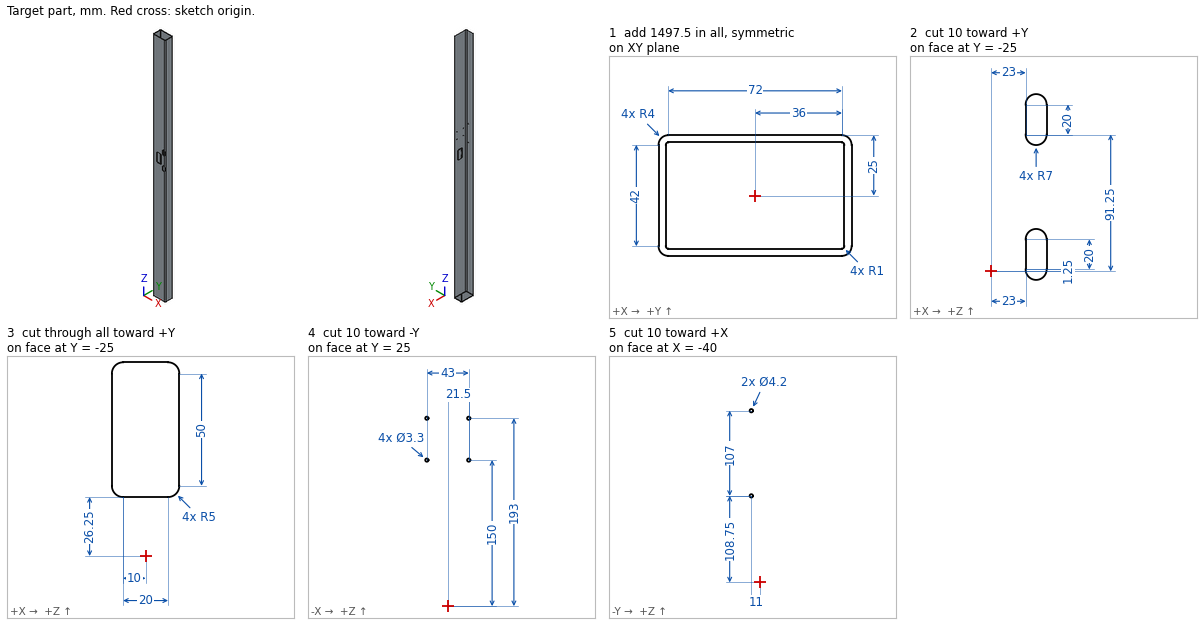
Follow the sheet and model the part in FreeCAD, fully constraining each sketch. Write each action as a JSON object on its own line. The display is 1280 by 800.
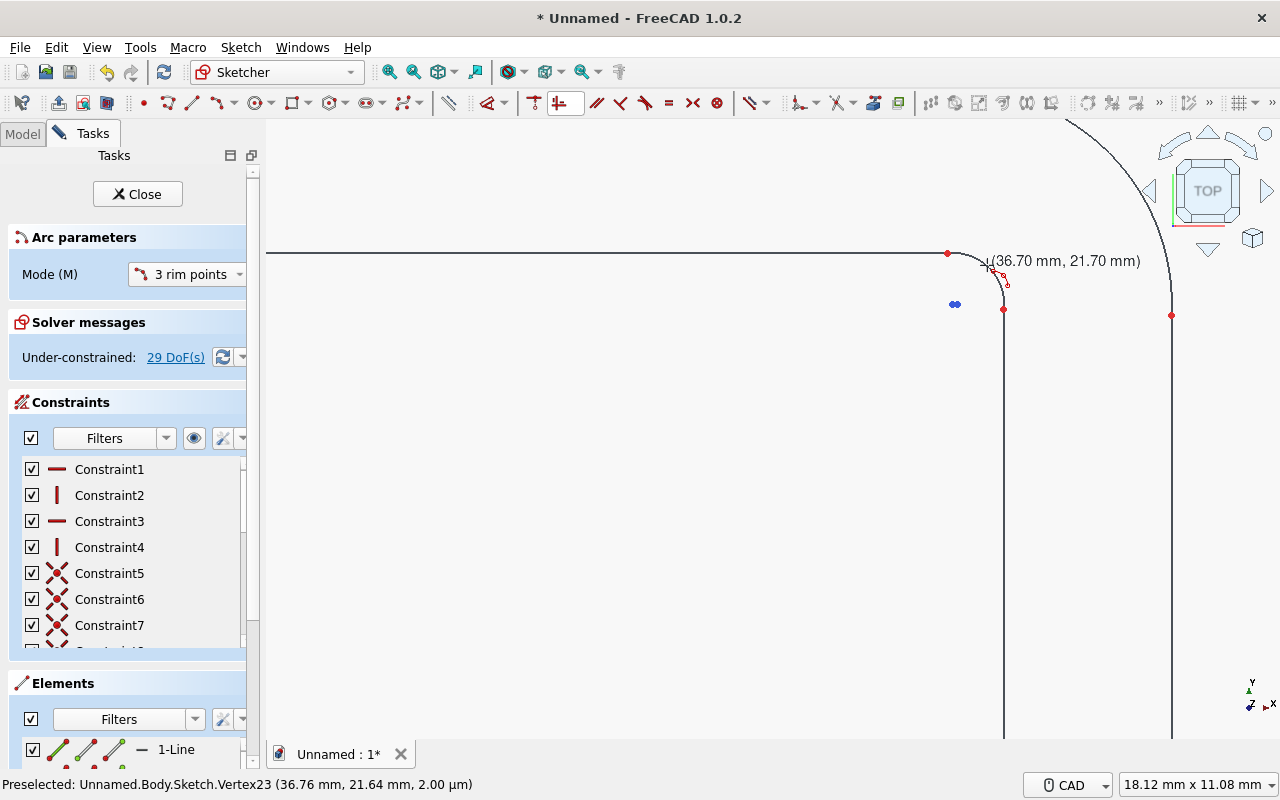
{"action": "scroll", "coordinate": [982, 264], "scroll_direction": "down", "scroll_amount": 10}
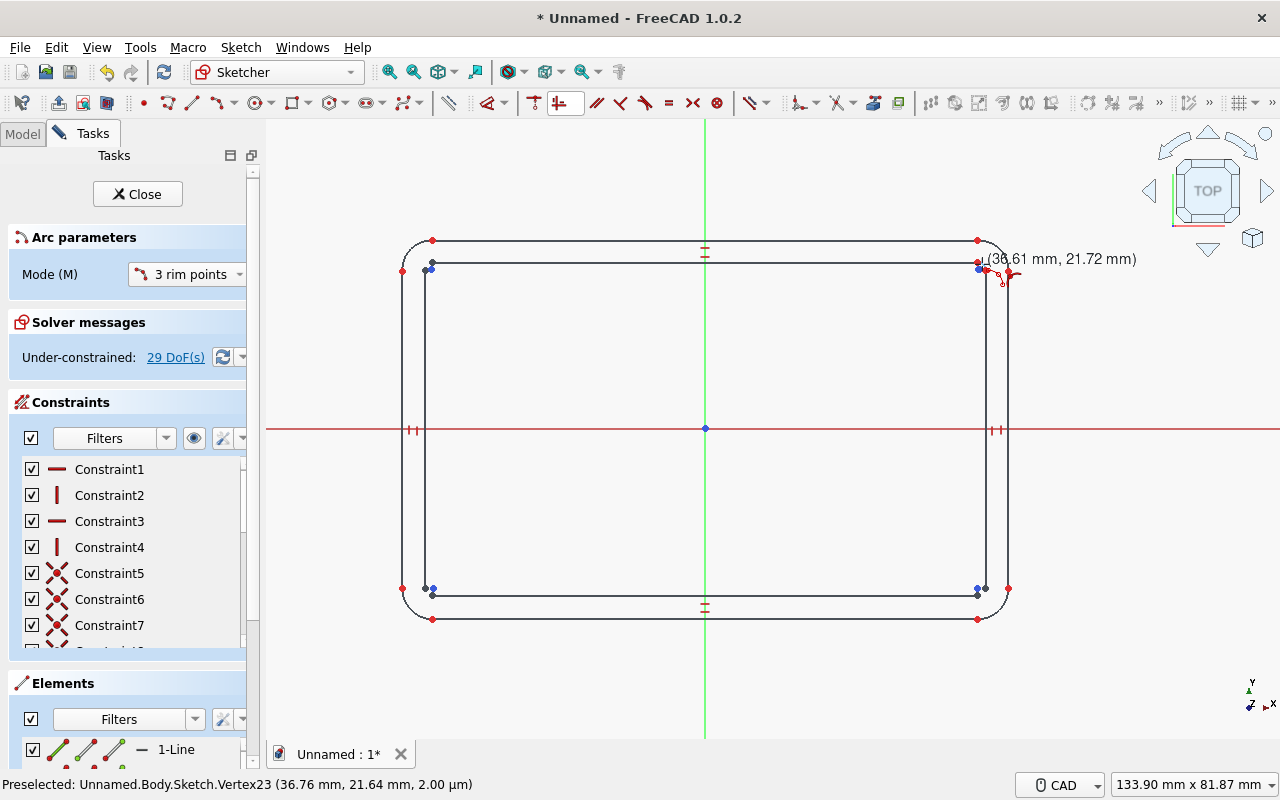
{"action": "scroll", "coordinate": [986, 588], "scroll_direction": "up", "scroll_amount": 4}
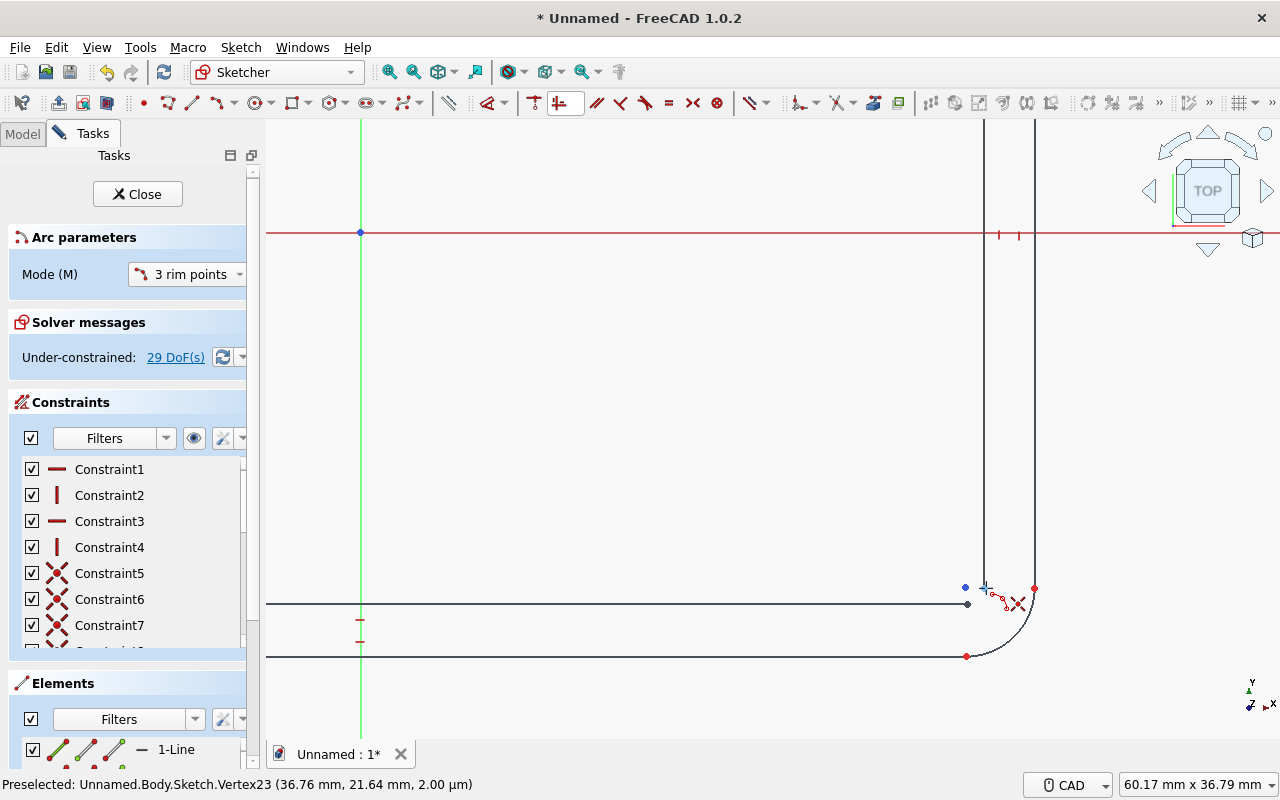
{"action": "left_click", "coordinate": [984, 588]}
{"action": "left_click", "coordinate": [967, 604]}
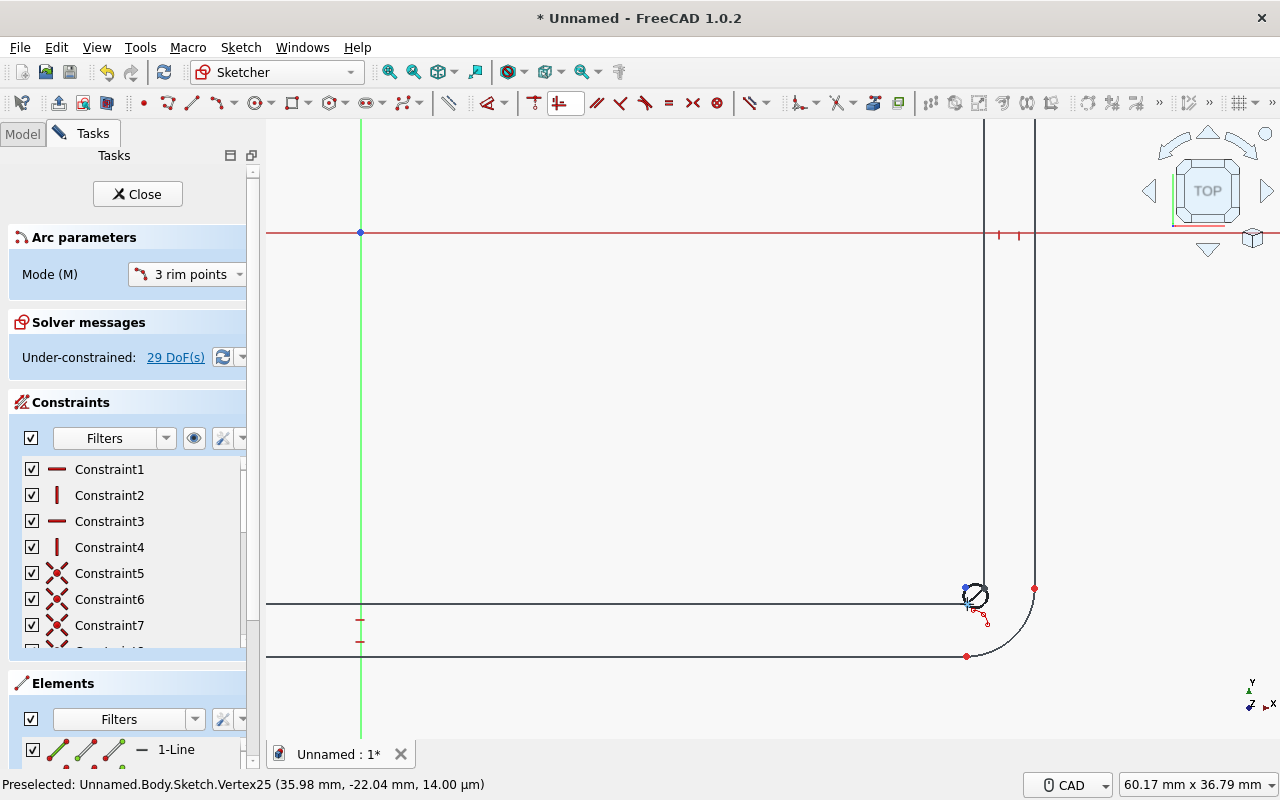
{"action": "scroll", "coordinate": [979, 599], "scroll_direction": "up", "scroll_amount": 6}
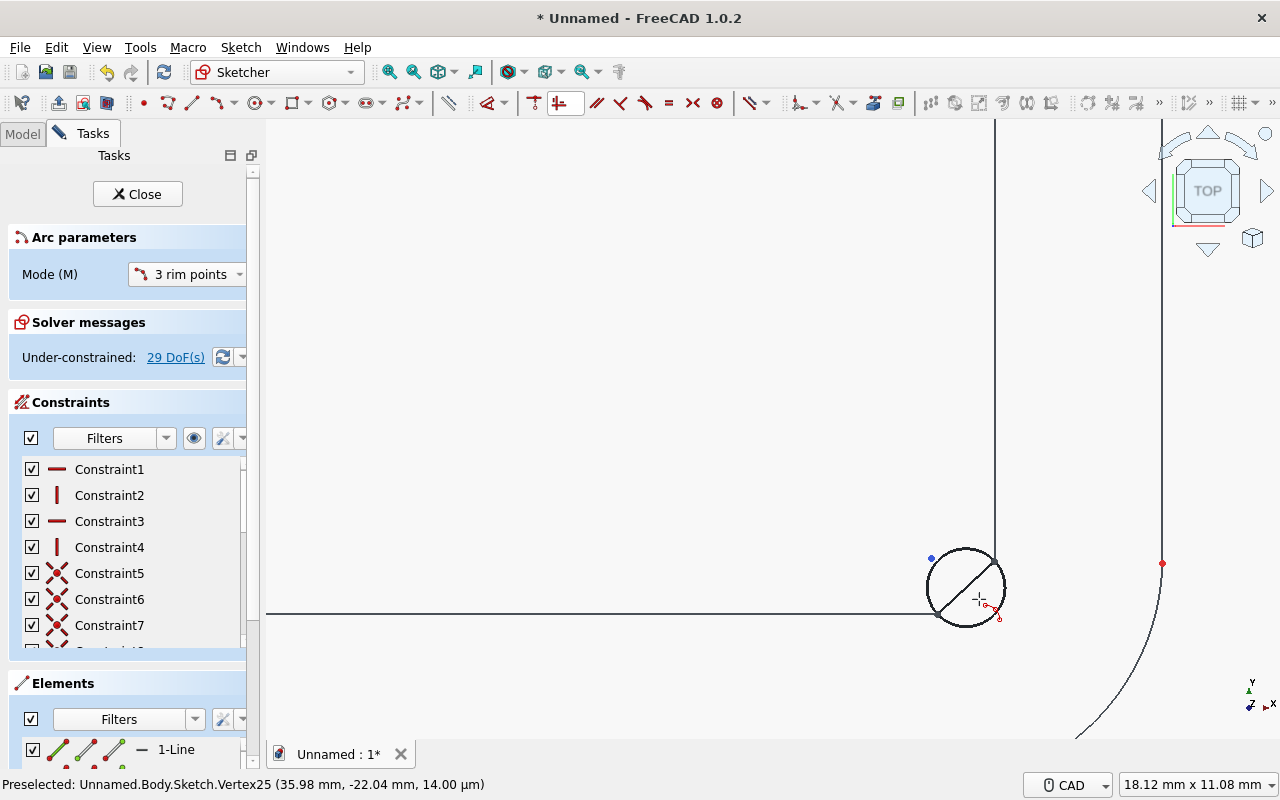
{"action": "left_click", "coordinate": [978, 596]}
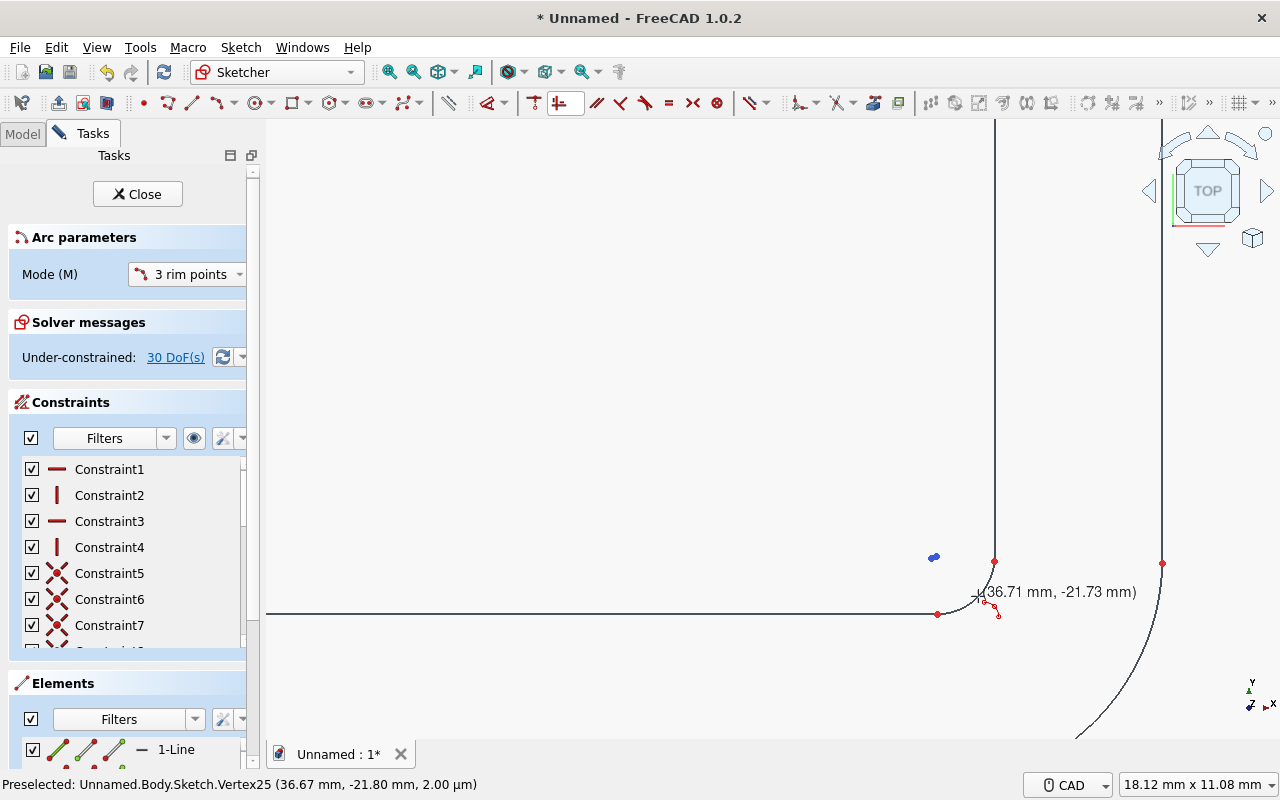
{"action": "scroll", "coordinate": [983, 593], "scroll_direction": "down", "scroll_amount": 10}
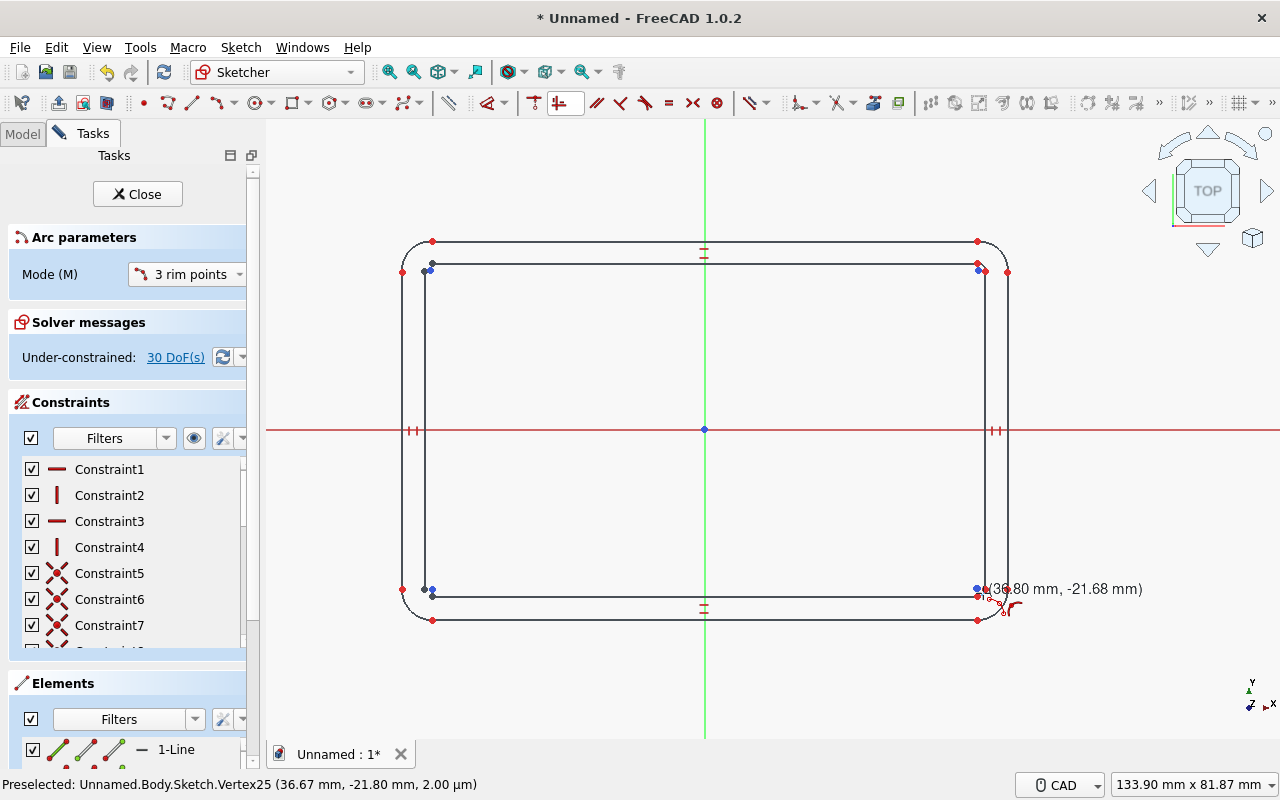
{"action": "scroll", "coordinate": [432, 596], "scroll_direction": "up", "scroll_amount": 4}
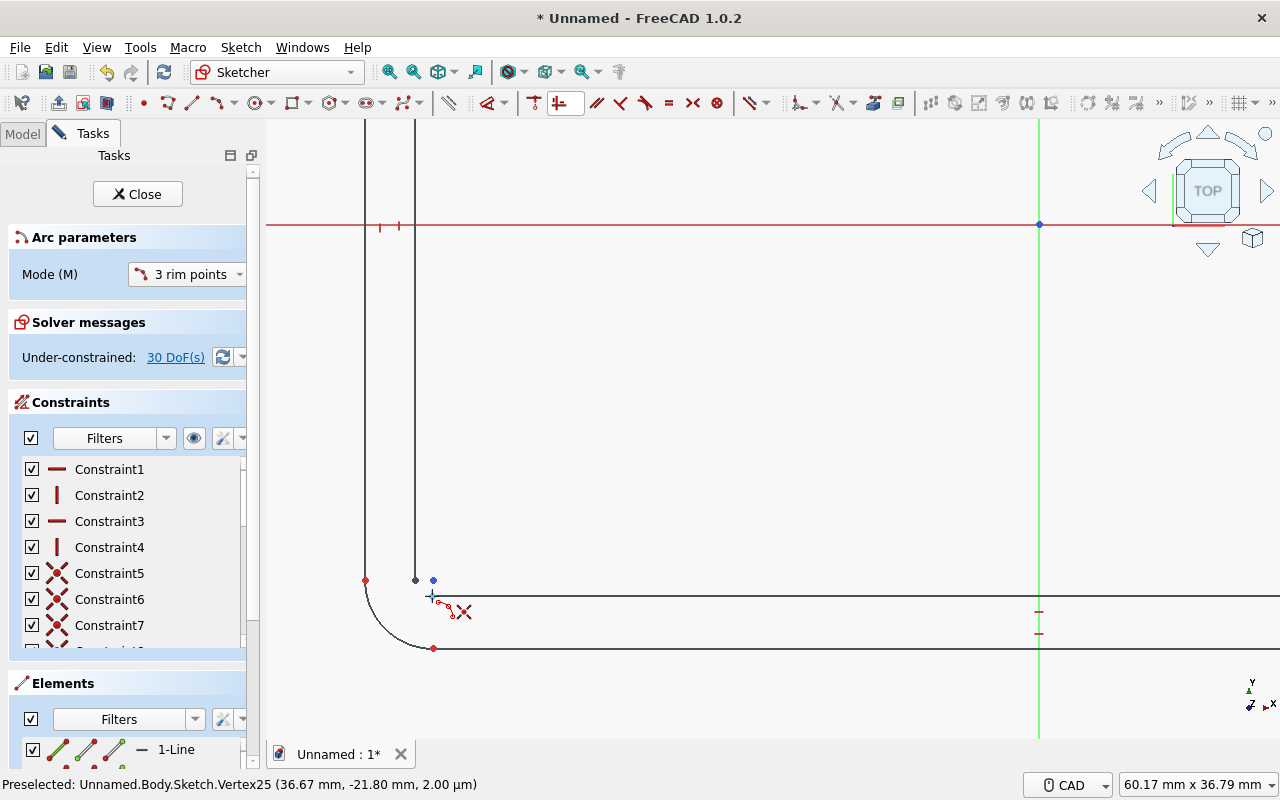
{"action": "left_click", "coordinate": [432, 596]}
{"action": "left_click", "coordinate": [415, 580]}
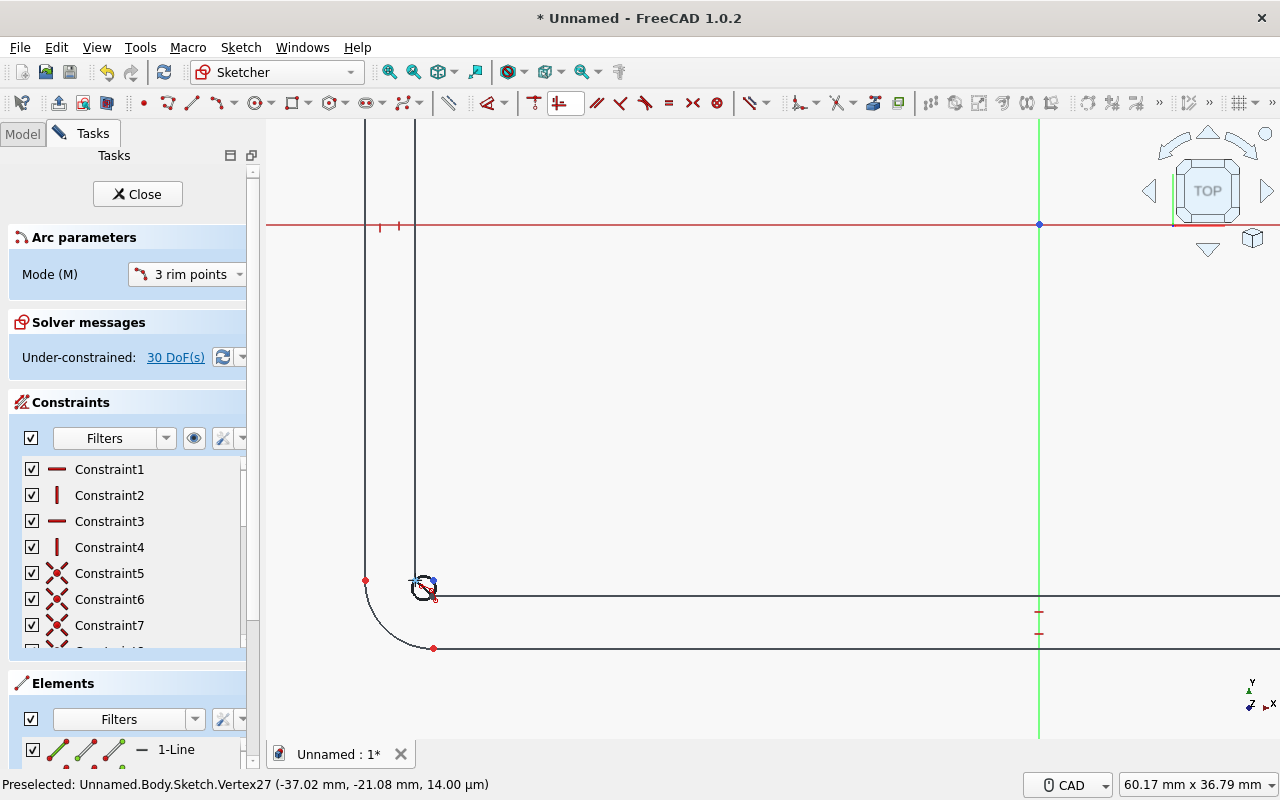
{"action": "scroll", "coordinate": [421, 591], "scroll_direction": "up", "scroll_amount": 6}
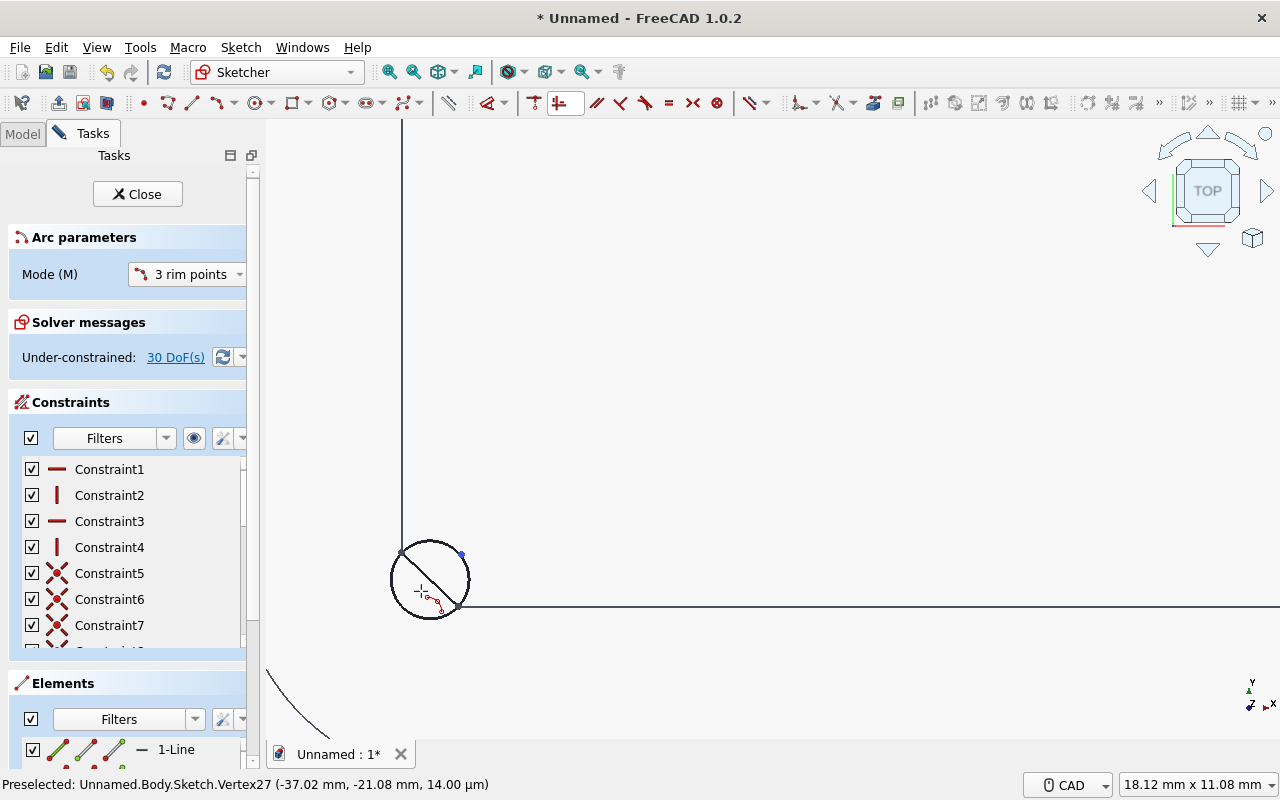
{"action": "left_click", "coordinate": [420, 588]}